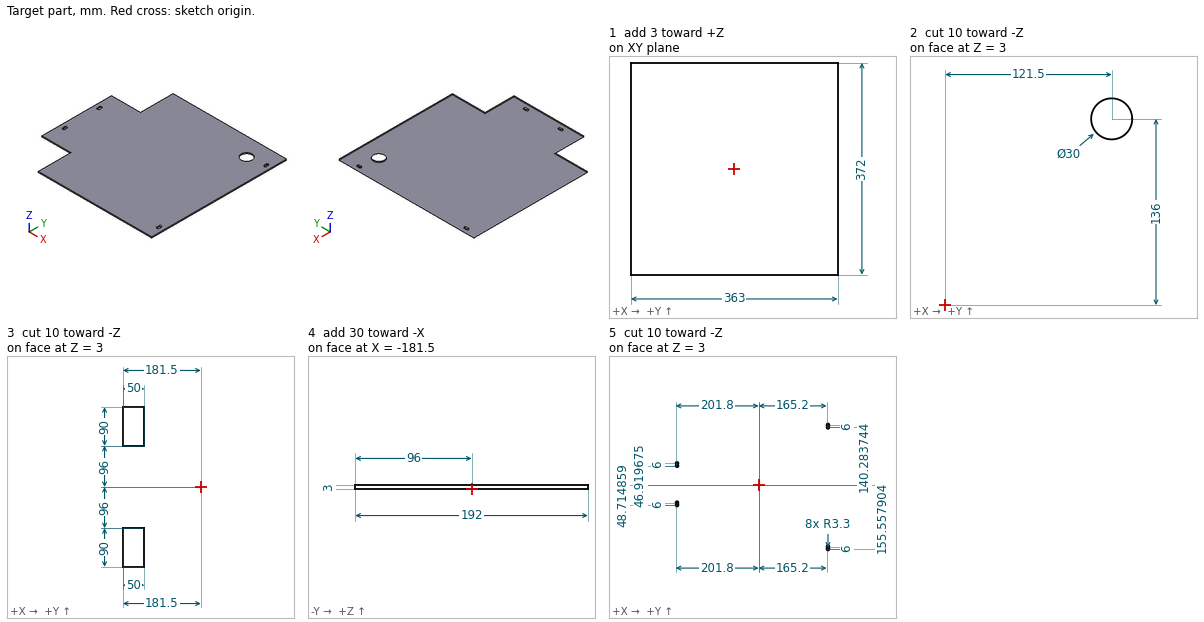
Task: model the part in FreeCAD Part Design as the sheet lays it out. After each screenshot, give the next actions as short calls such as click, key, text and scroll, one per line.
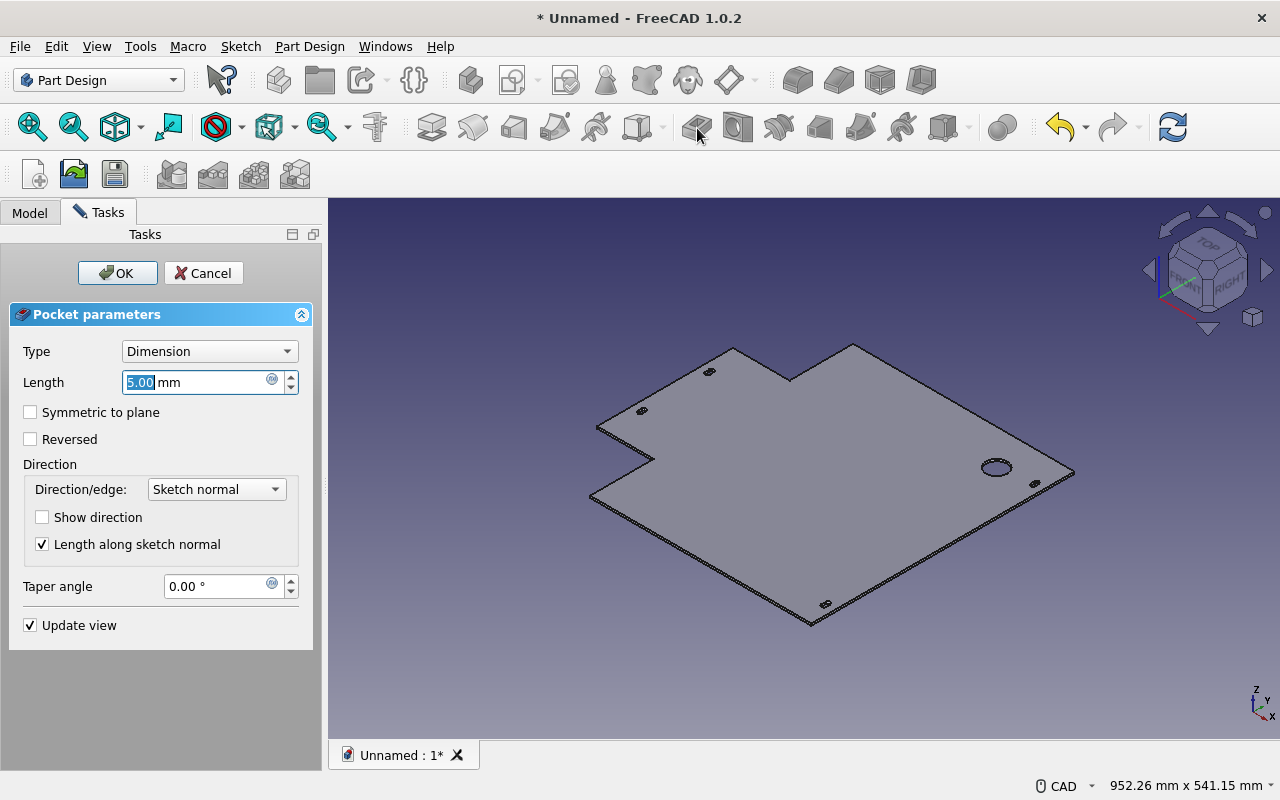
text(10)
key(Tab)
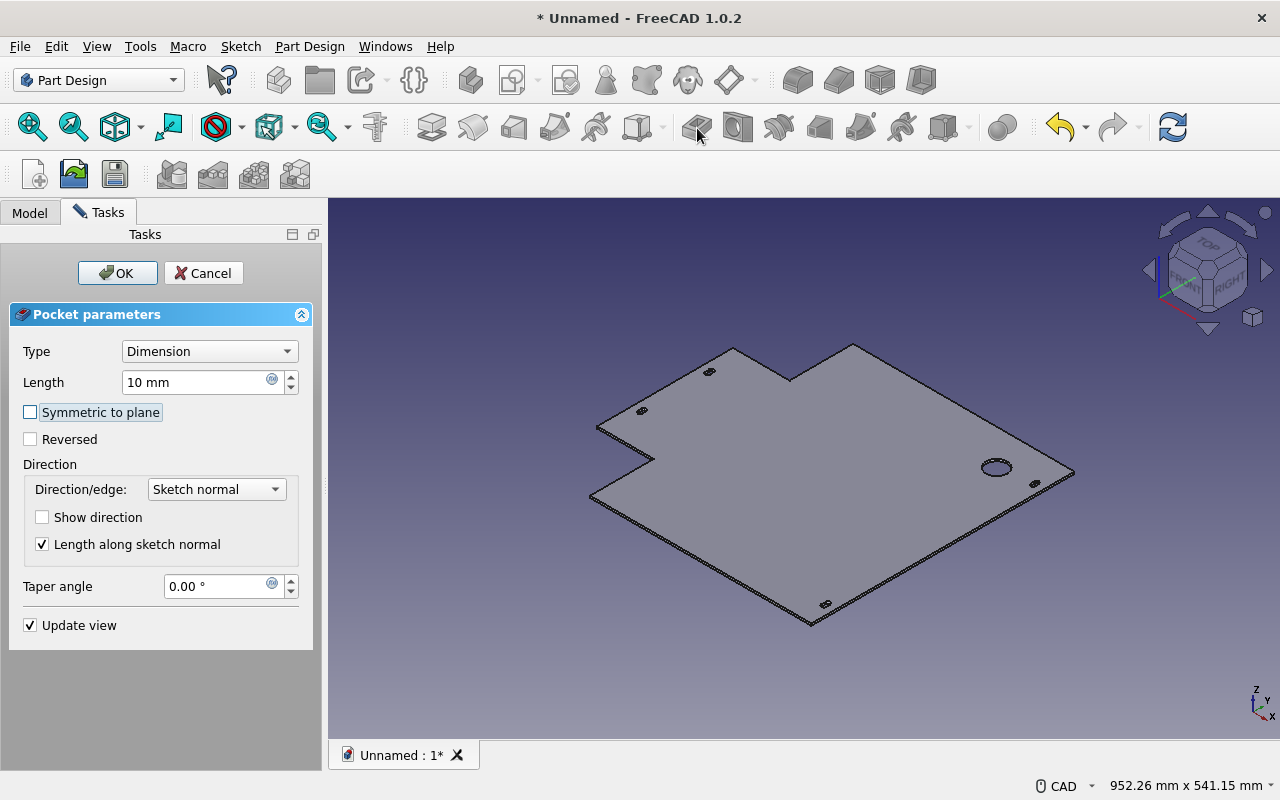
click(118, 273)